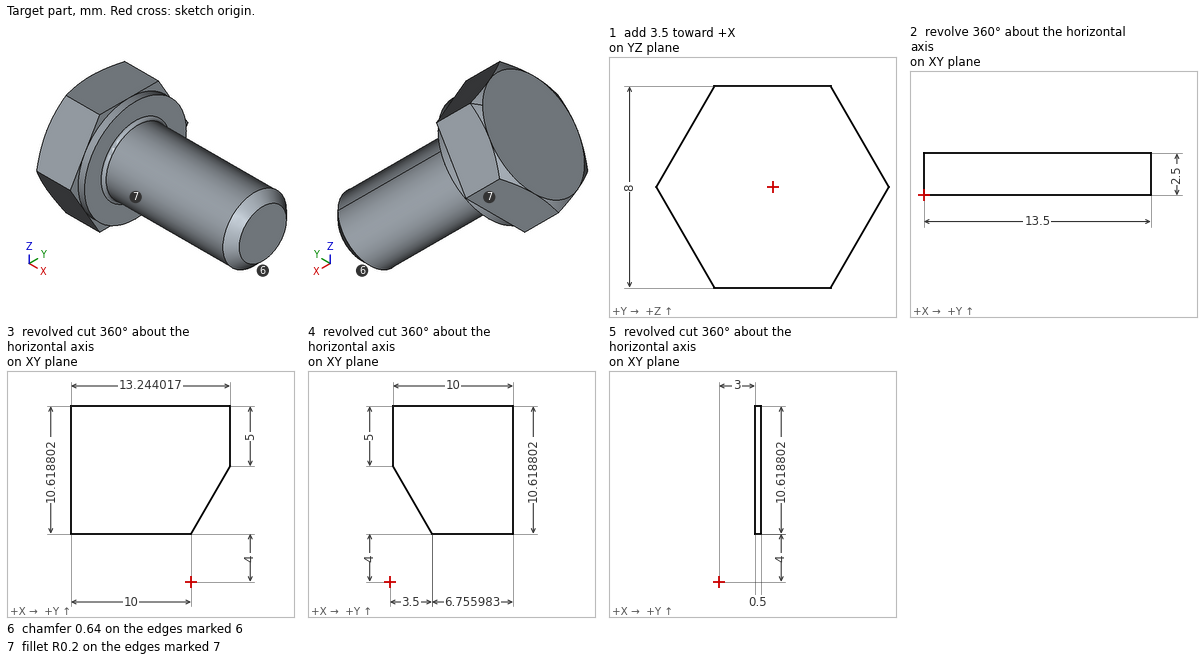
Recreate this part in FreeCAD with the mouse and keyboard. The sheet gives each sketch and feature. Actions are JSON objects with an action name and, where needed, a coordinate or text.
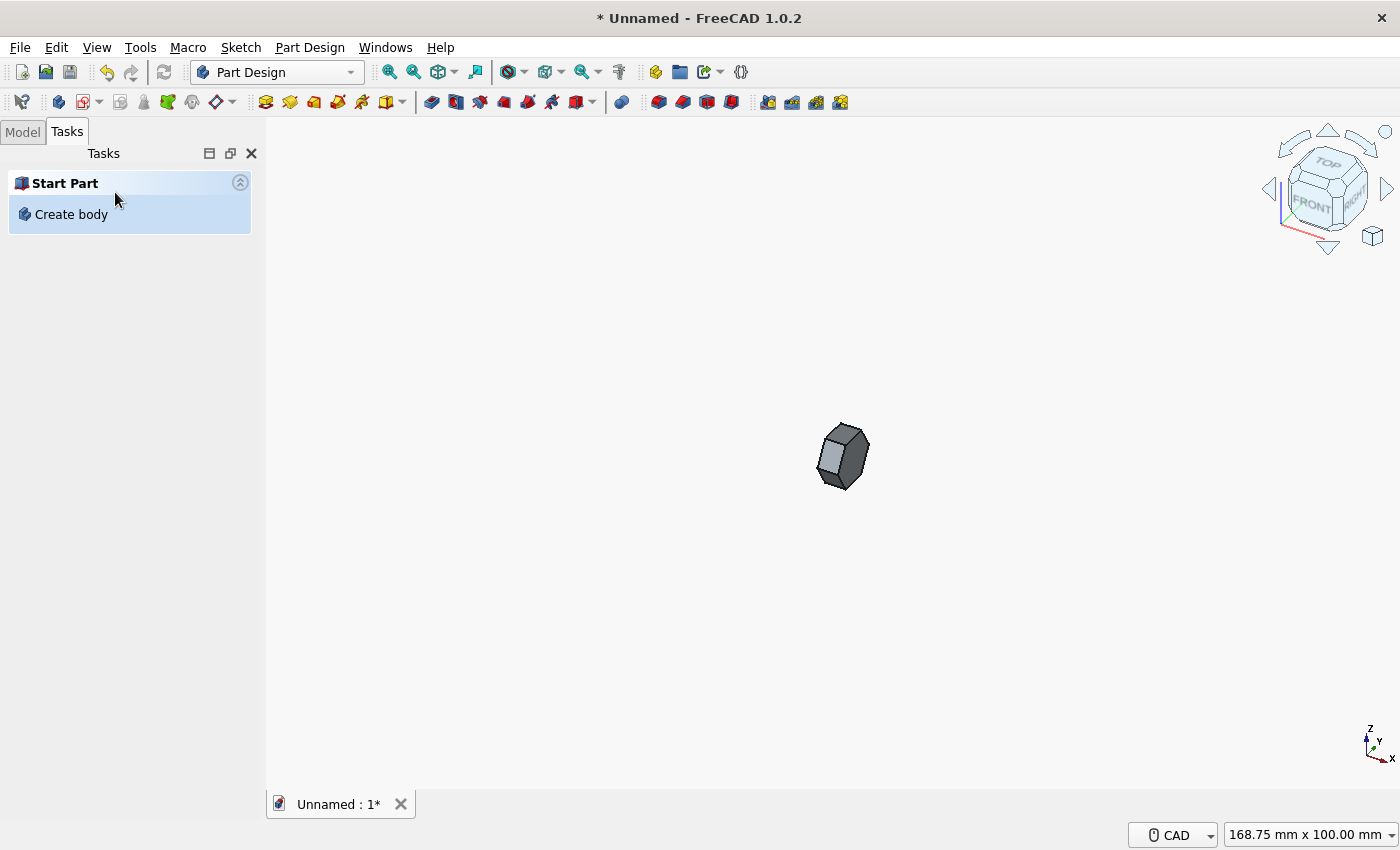
{"action": "left_click", "coordinate": [390, 72]}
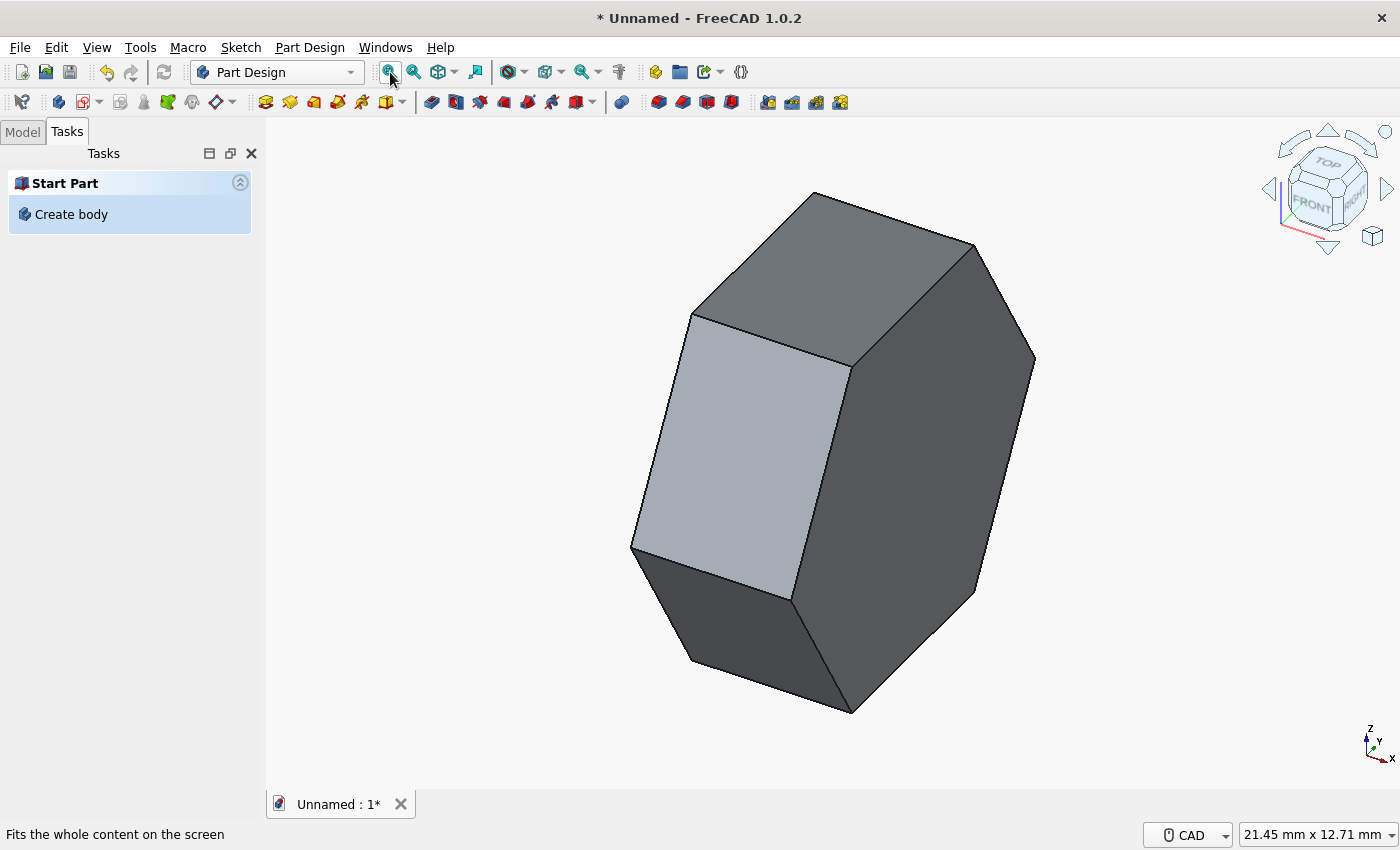
{"action": "left_click", "coordinate": [84, 102]}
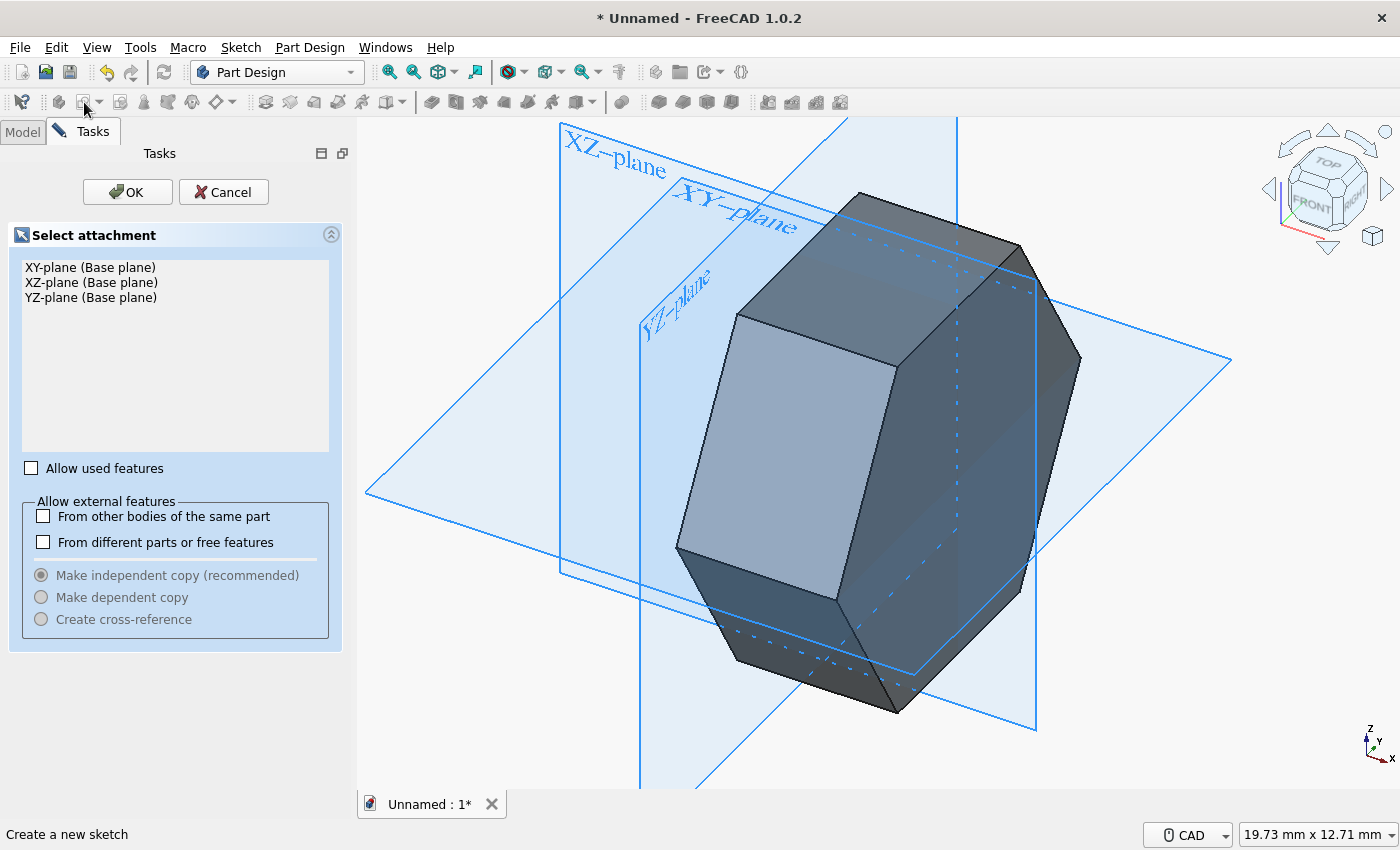
{"action": "left_click", "coordinate": [82, 268]}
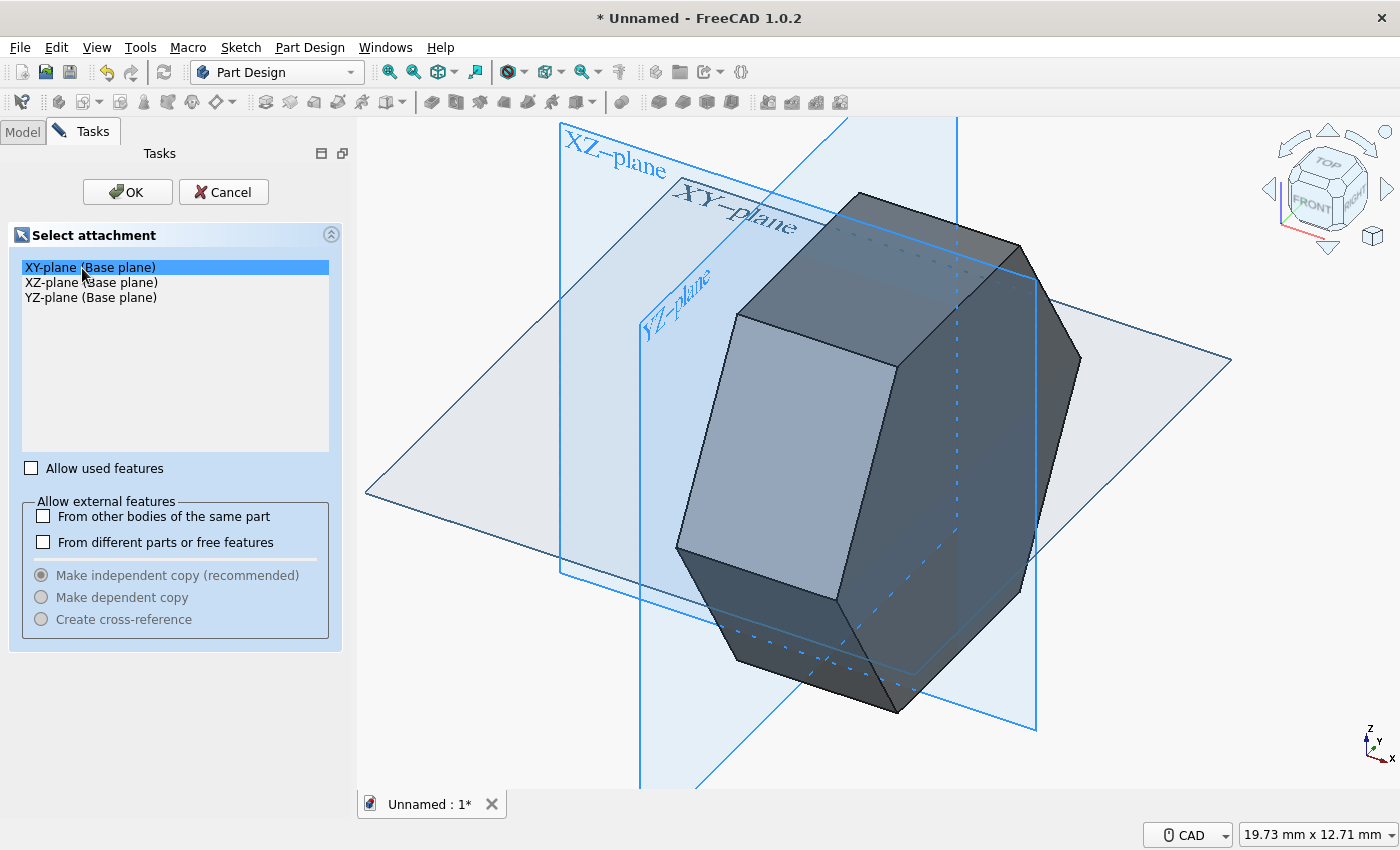
{"action": "left_click", "coordinate": [128, 192]}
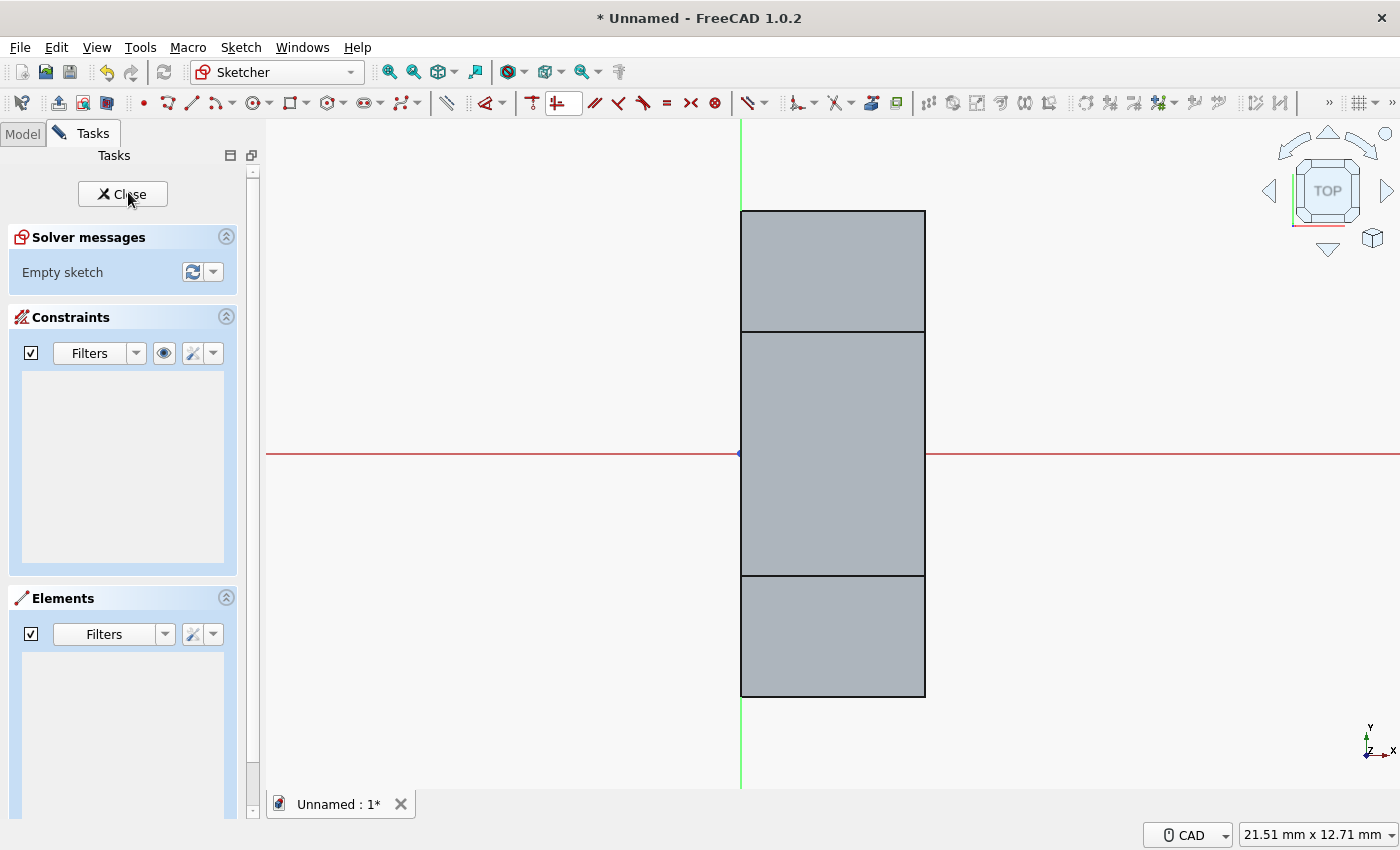
{"action": "left_click", "coordinate": [108, 104]}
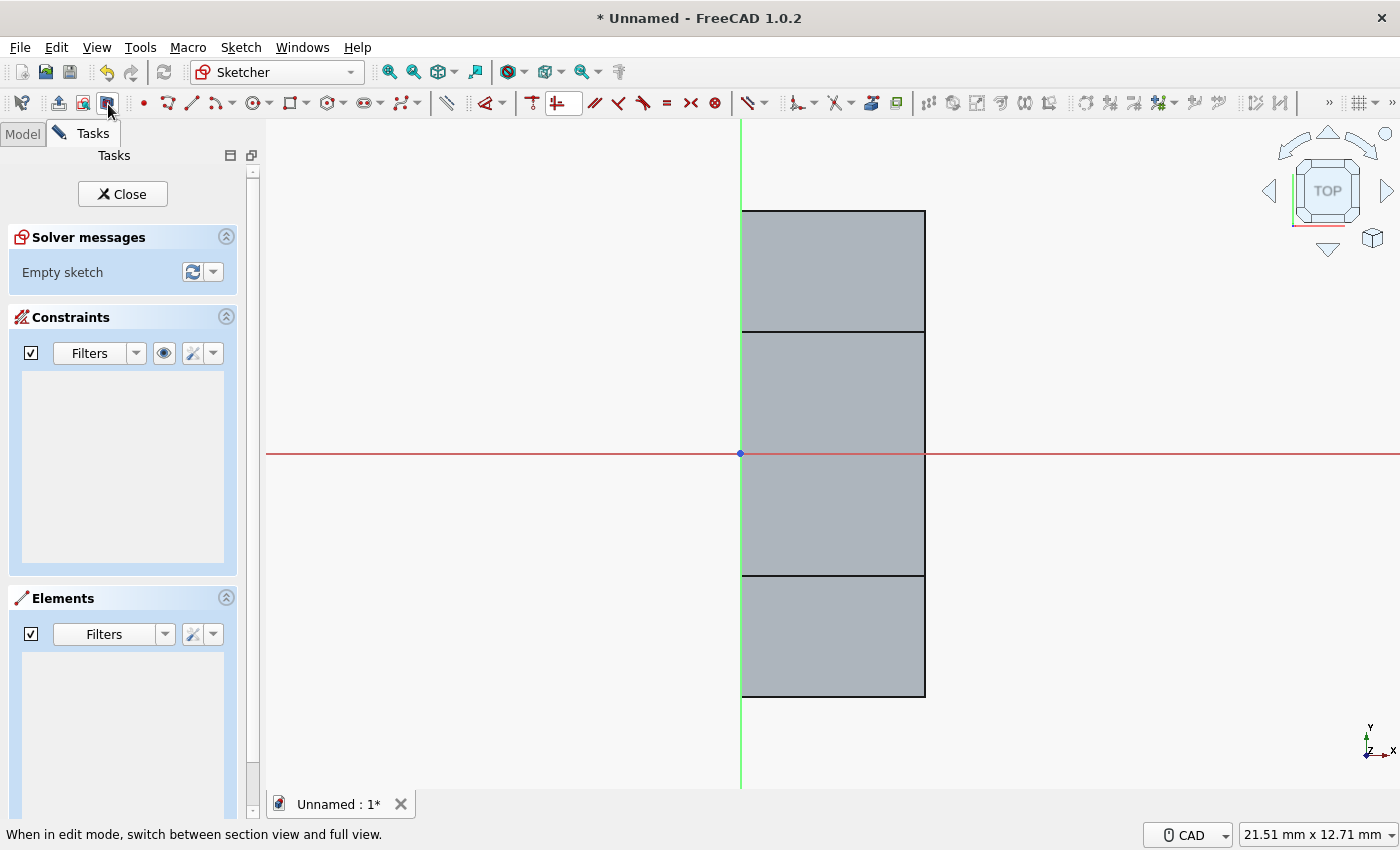
{"action": "scroll", "coordinate": [294, 588], "scroll_direction": "down", "scroll_amount": 2}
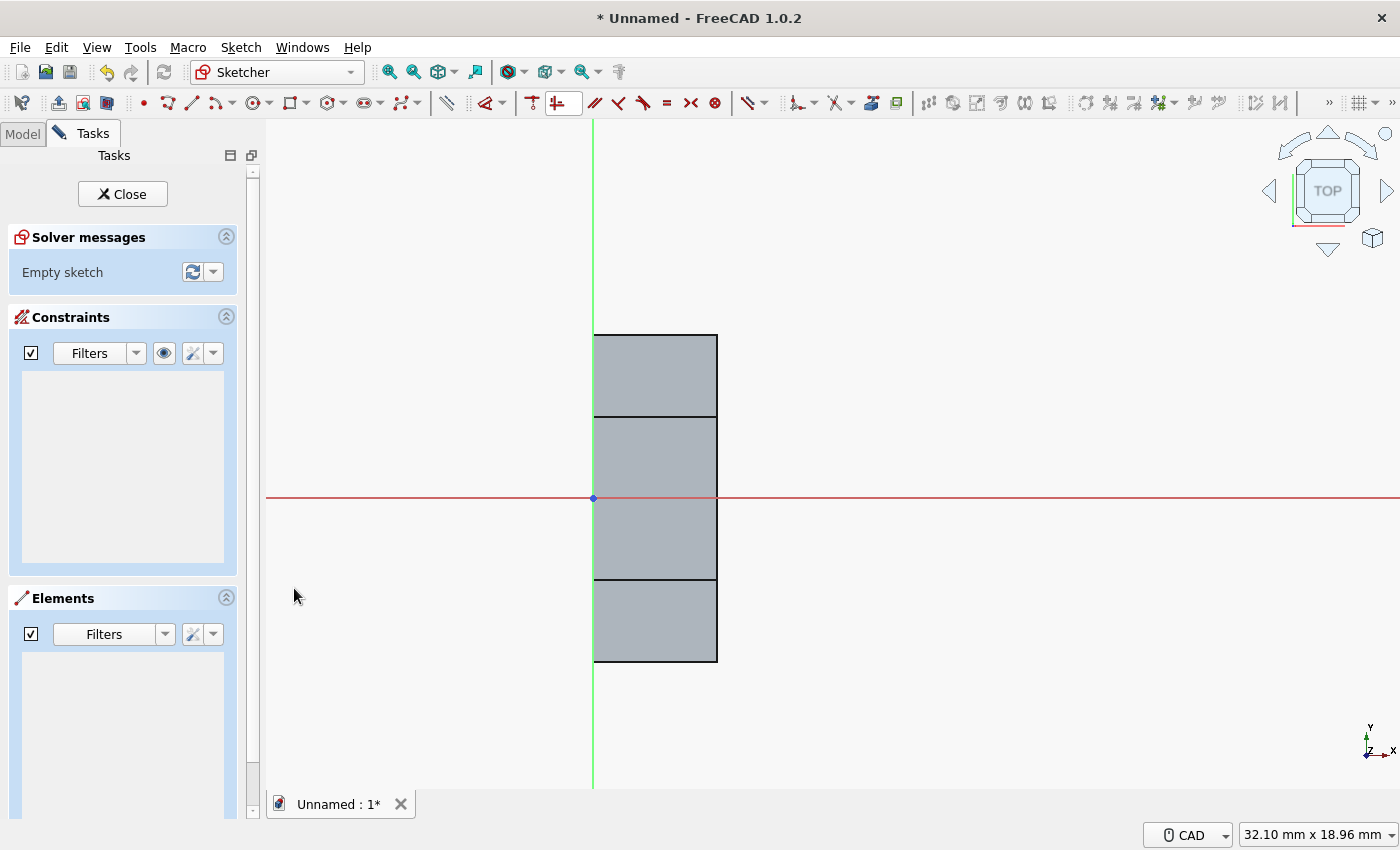
{"action": "scroll", "coordinate": [969, 455], "scroll_direction": "up", "scroll_amount": 2}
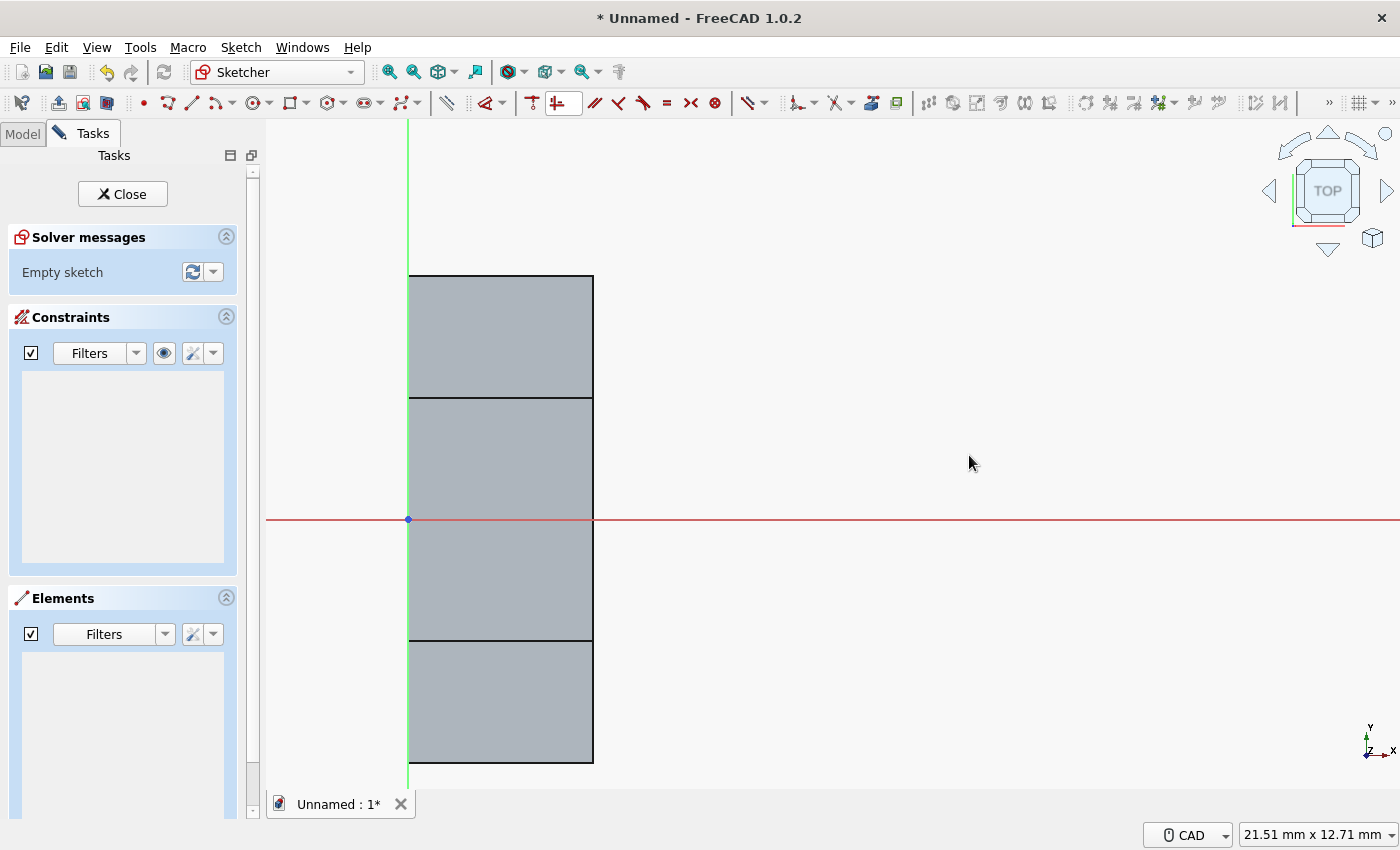
{"action": "left_click", "coordinate": [290, 104]}